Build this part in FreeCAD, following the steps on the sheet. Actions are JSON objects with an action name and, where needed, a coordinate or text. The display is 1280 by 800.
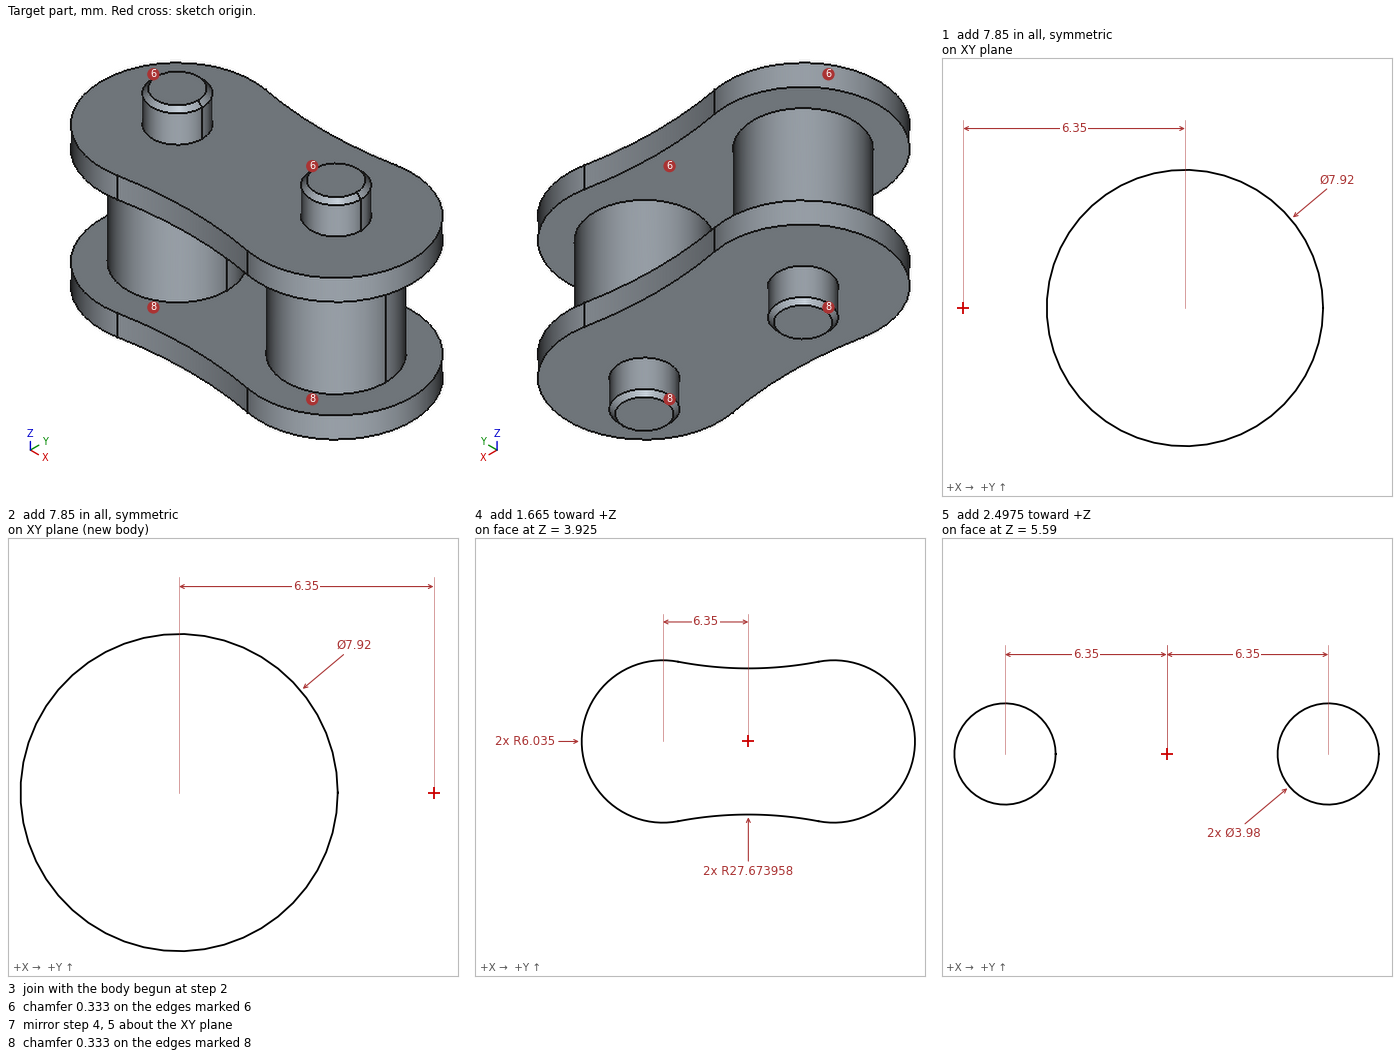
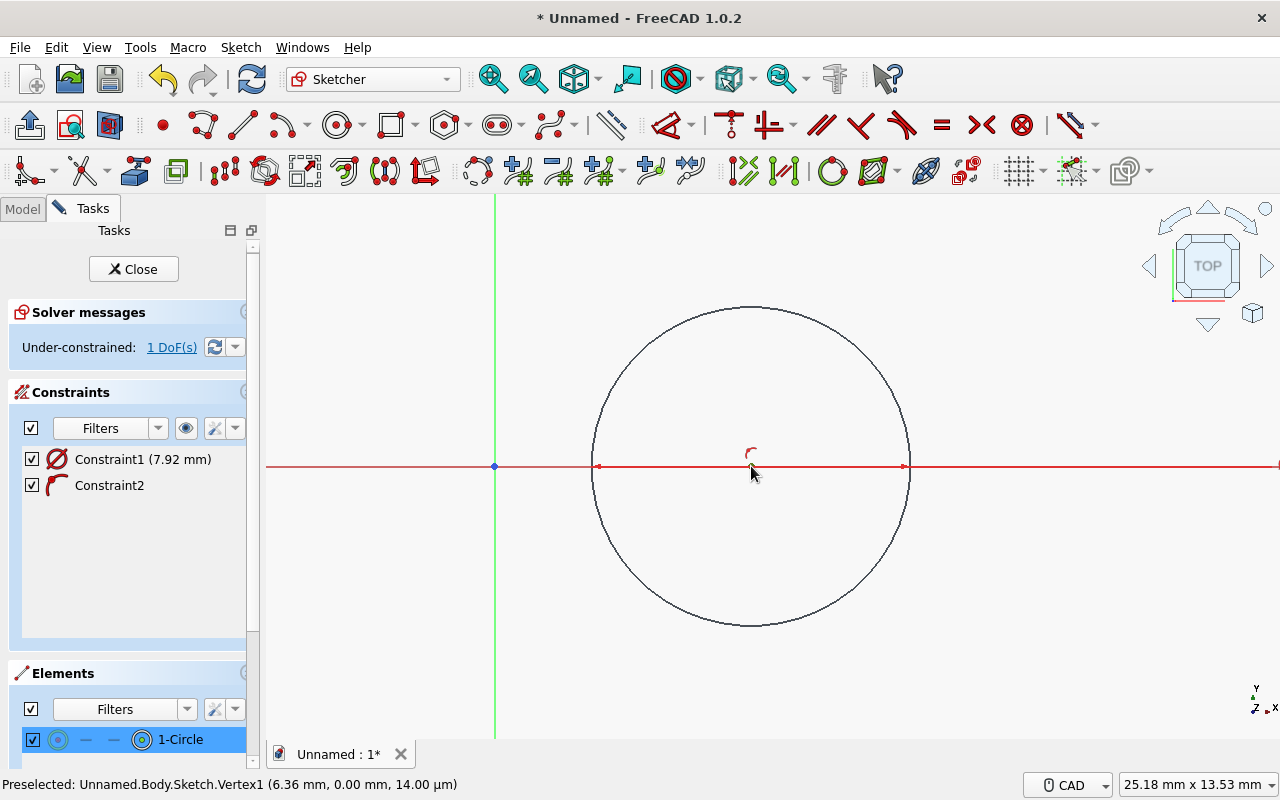
{"action": "left_click", "coordinate": [694, 126]}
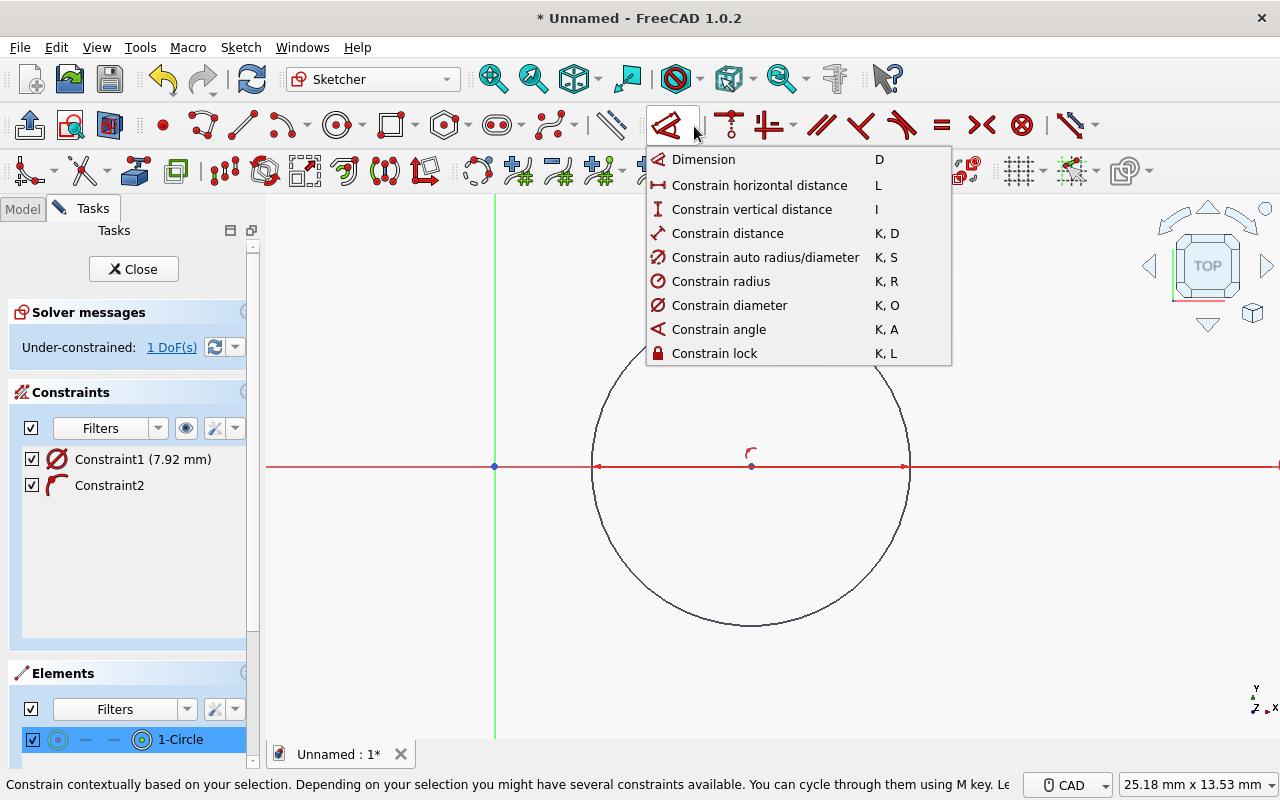
{"action": "left_click", "coordinate": [799, 185]}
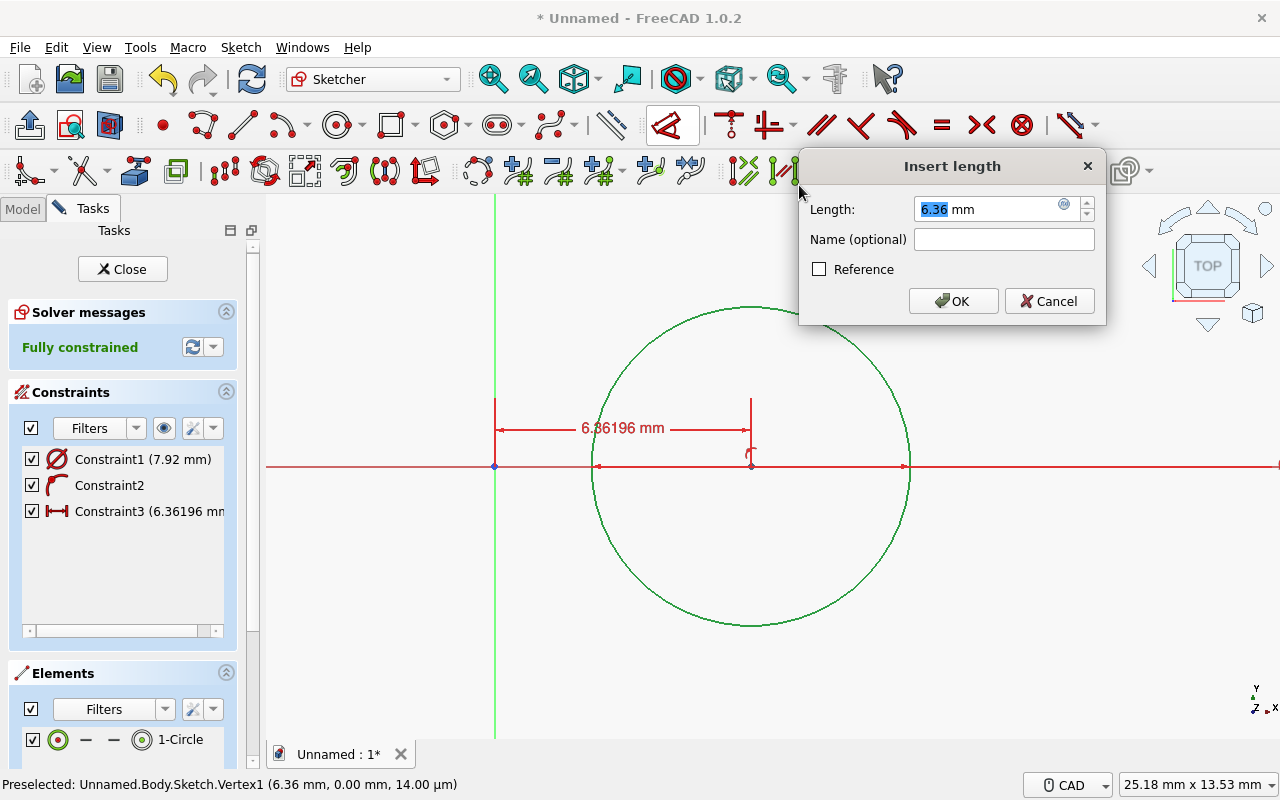
{"action": "type", "text": "6.35"}
{"action": "key", "text": "Return"}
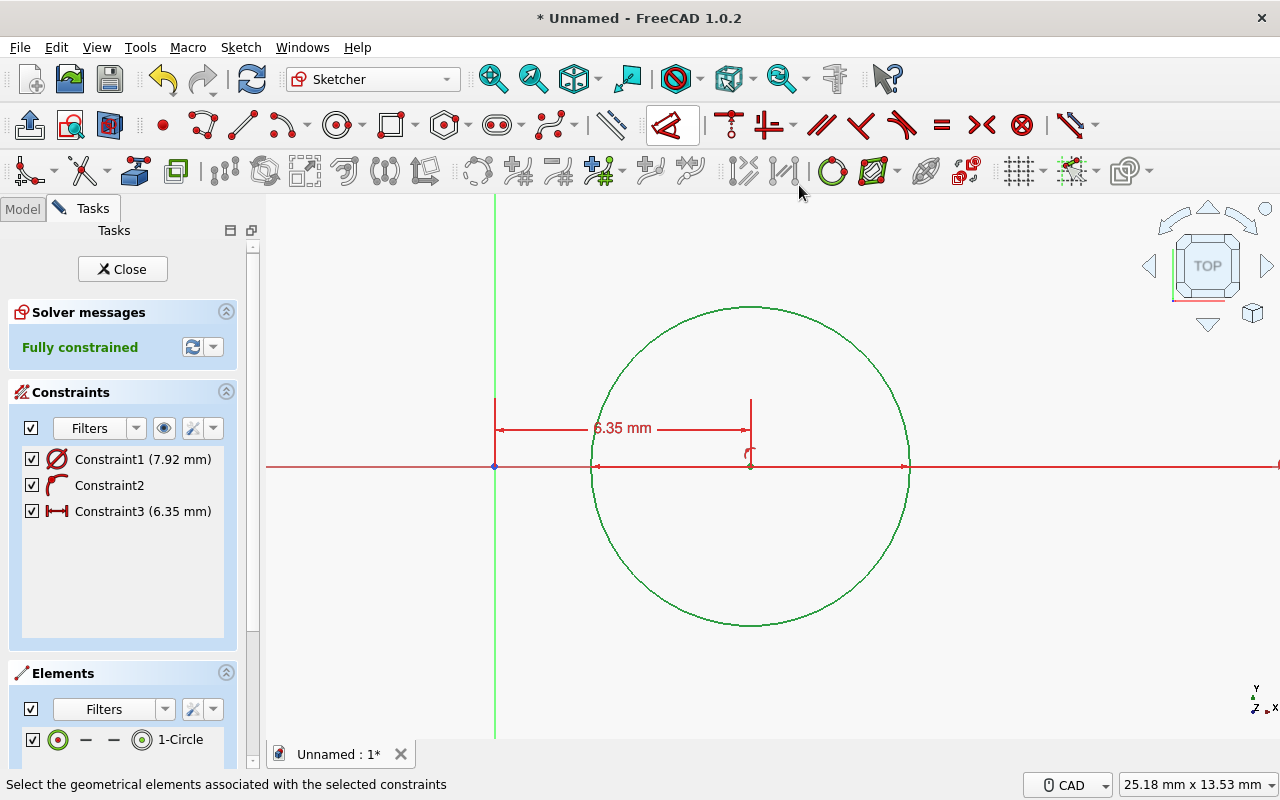
{"action": "left_click", "coordinate": [123, 269]}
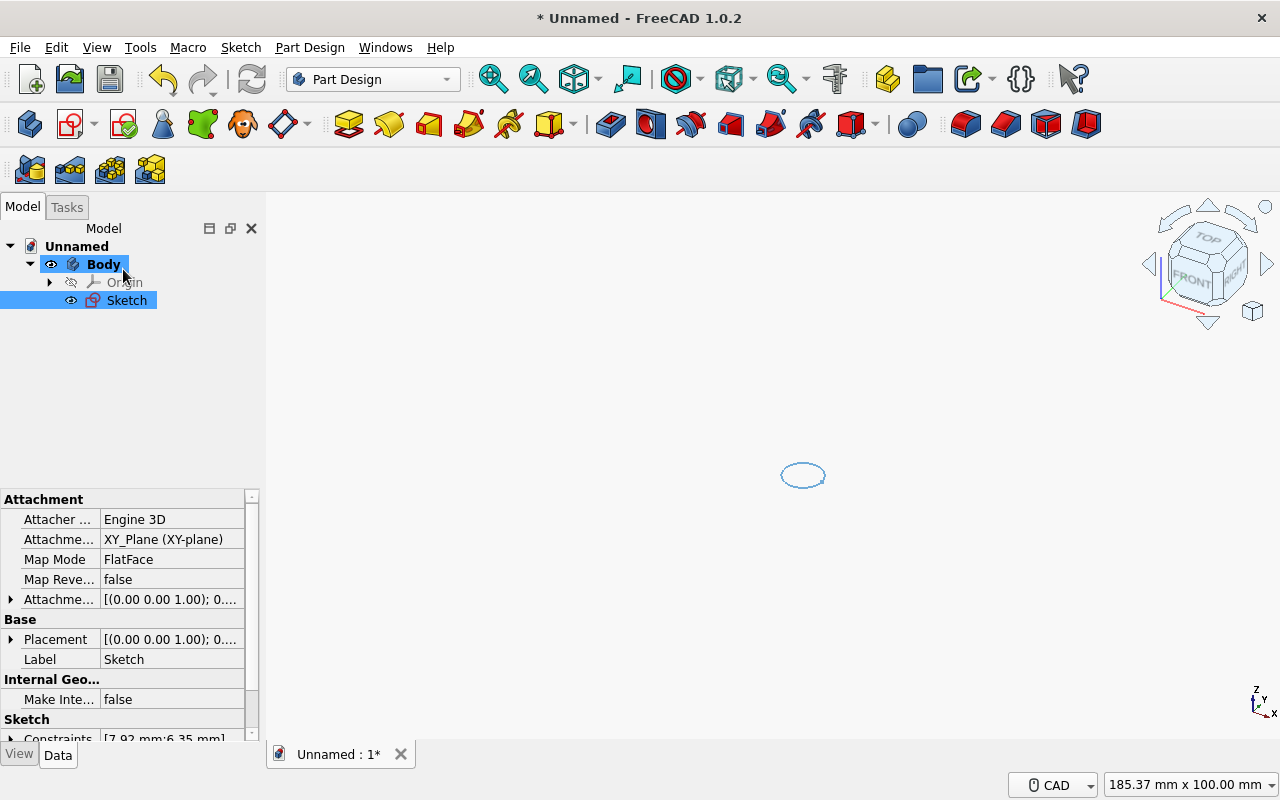
{"action": "left_click", "coordinate": [350, 124]}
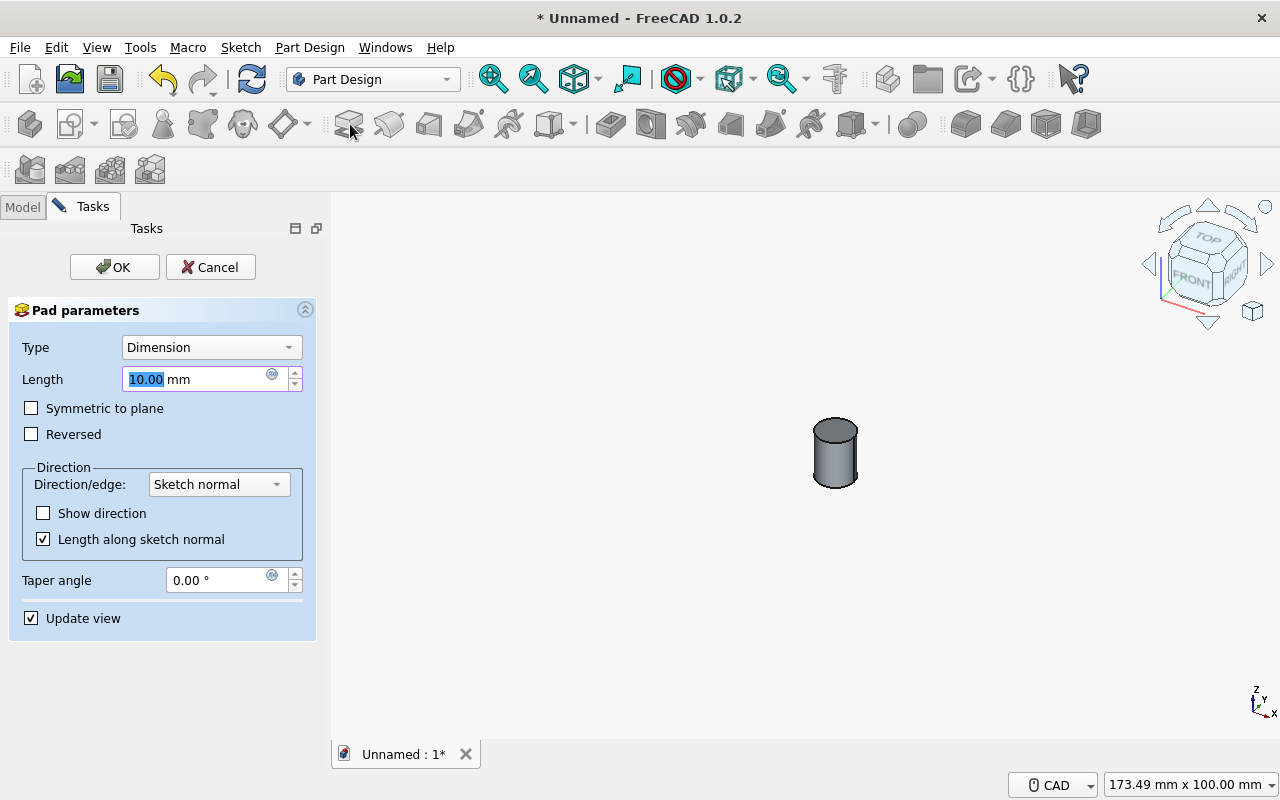
{"action": "type", "text": "7.85"}
{"action": "key", "text": "Tab"}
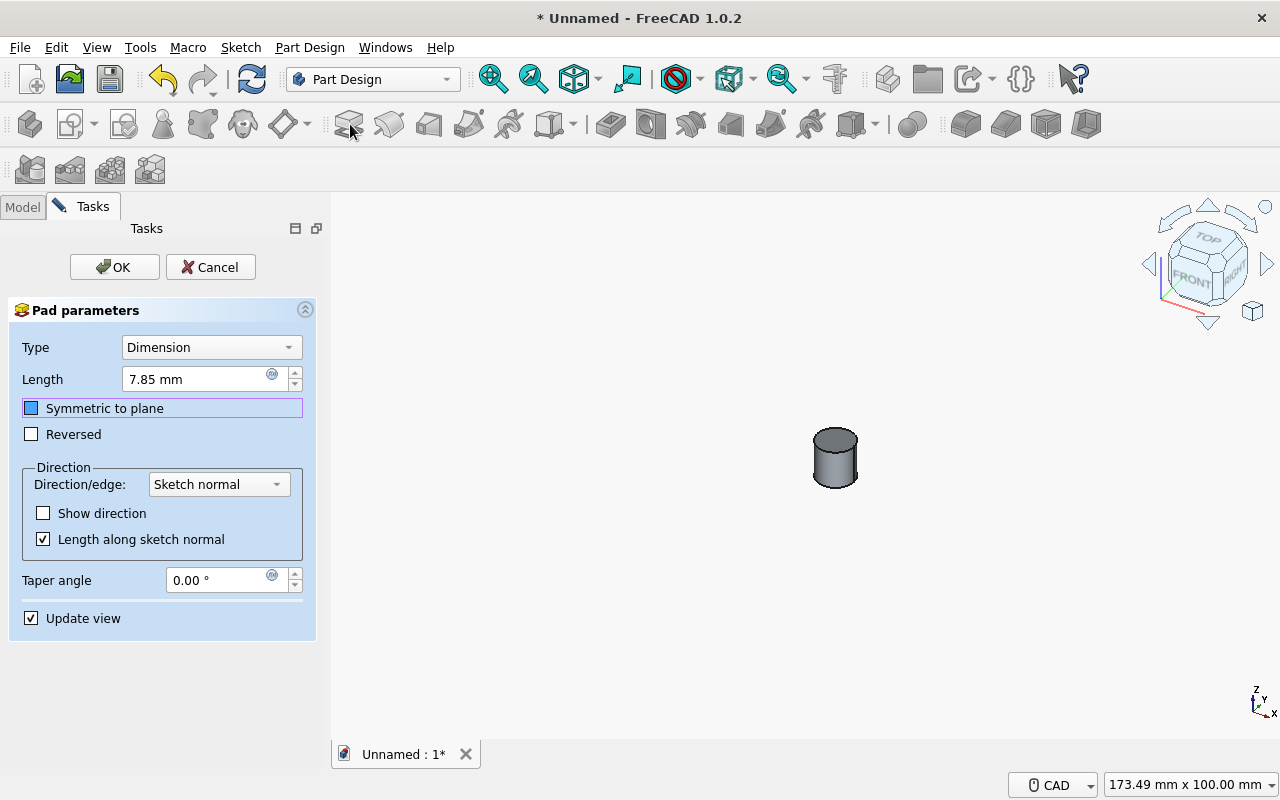
{"action": "left_click", "coordinate": [30, 408]}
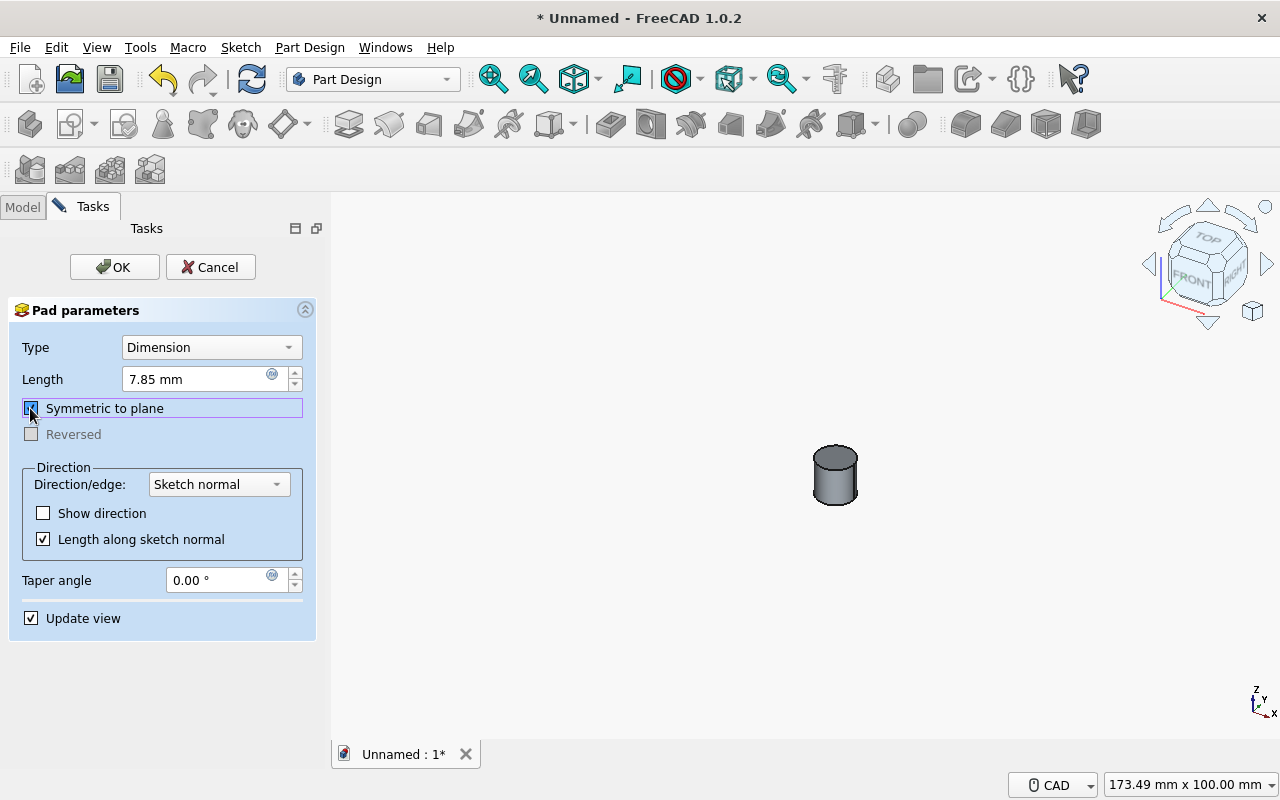
{"action": "left_click", "coordinate": [115, 267]}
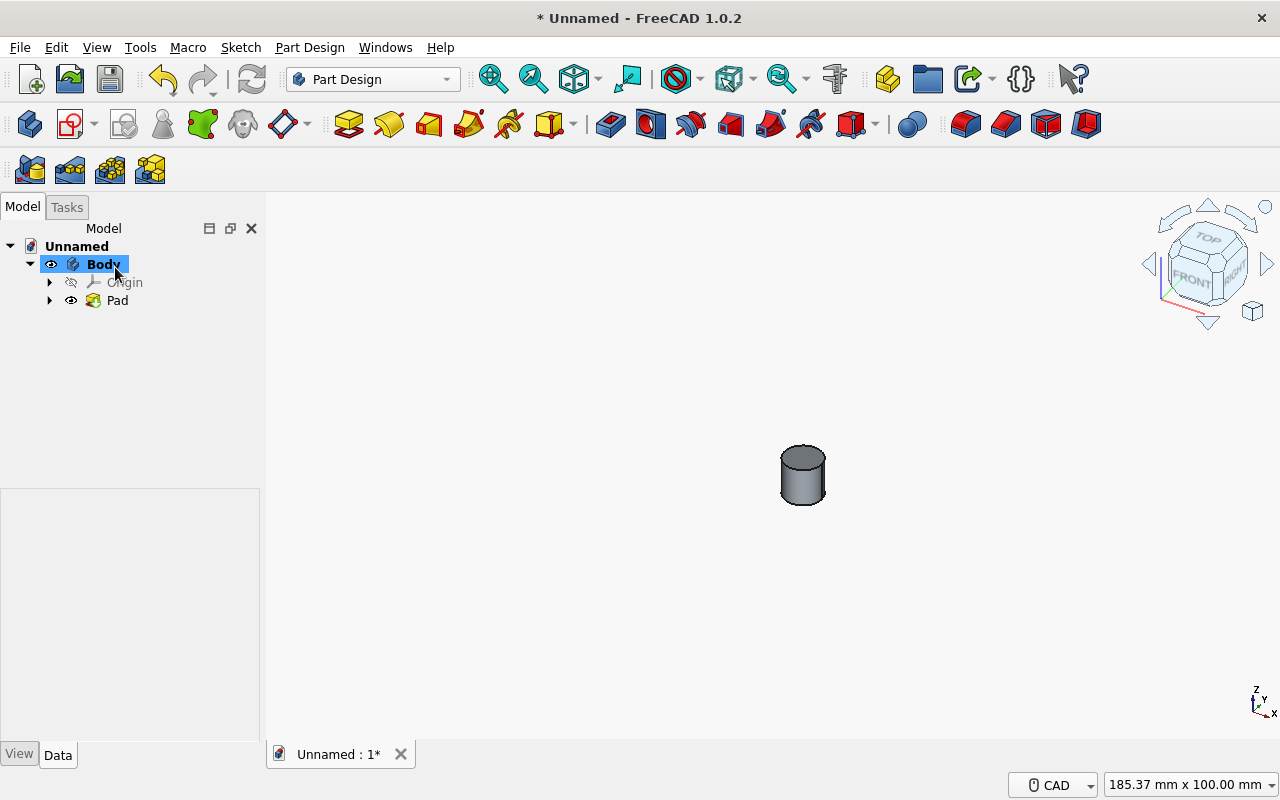
{"action": "left_click", "coordinate": [494, 80]}